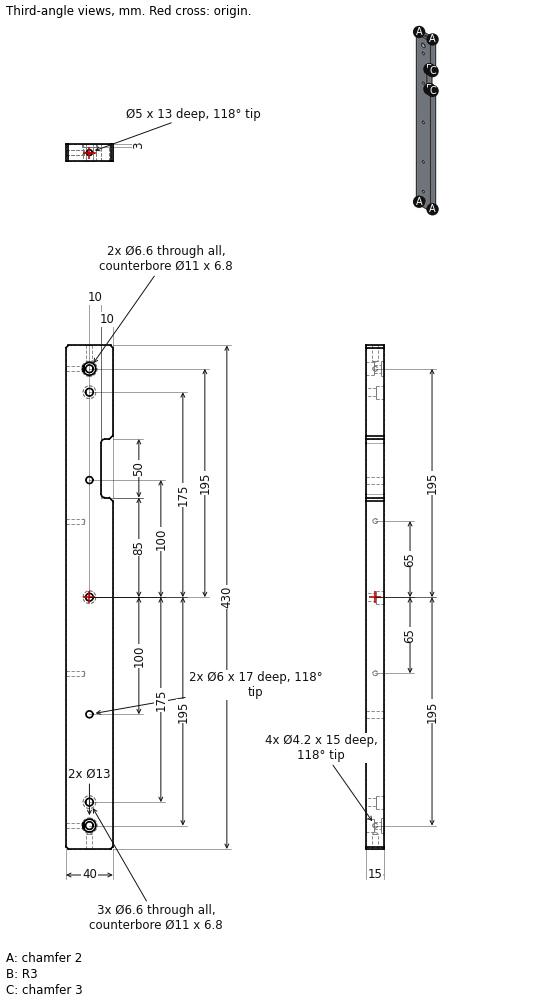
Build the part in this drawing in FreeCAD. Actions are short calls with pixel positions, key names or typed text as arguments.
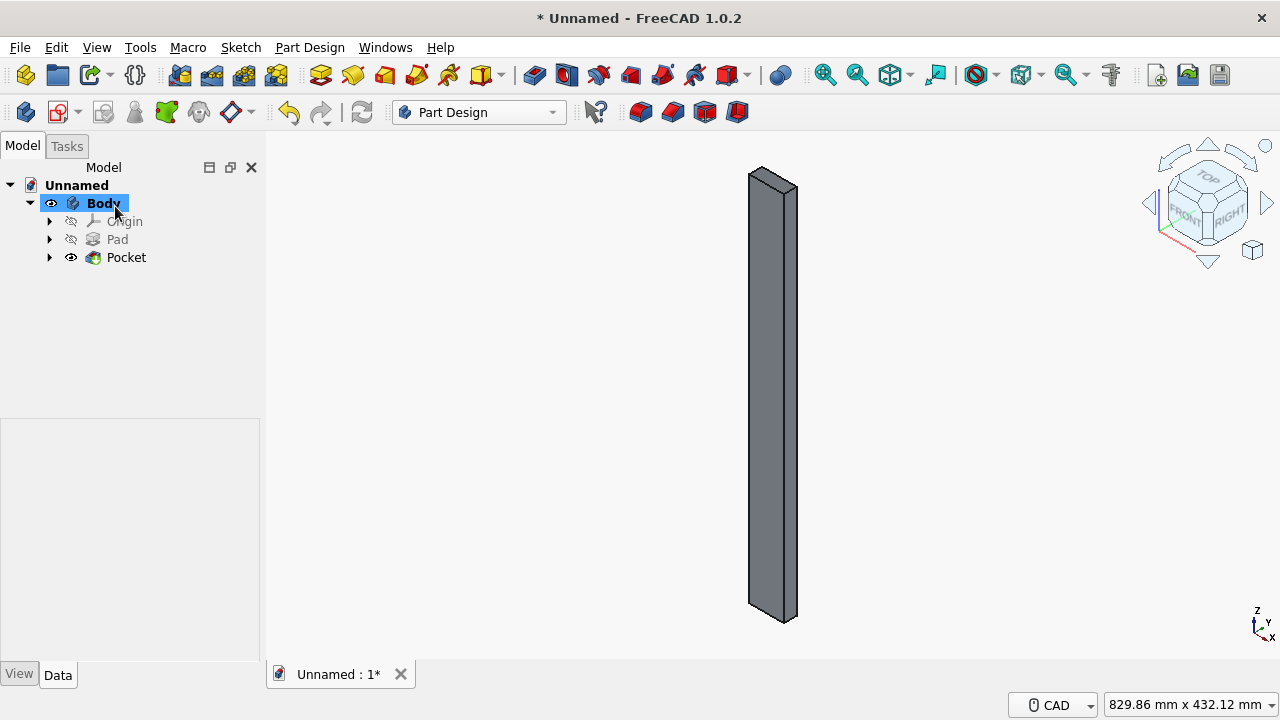
click(767, 214)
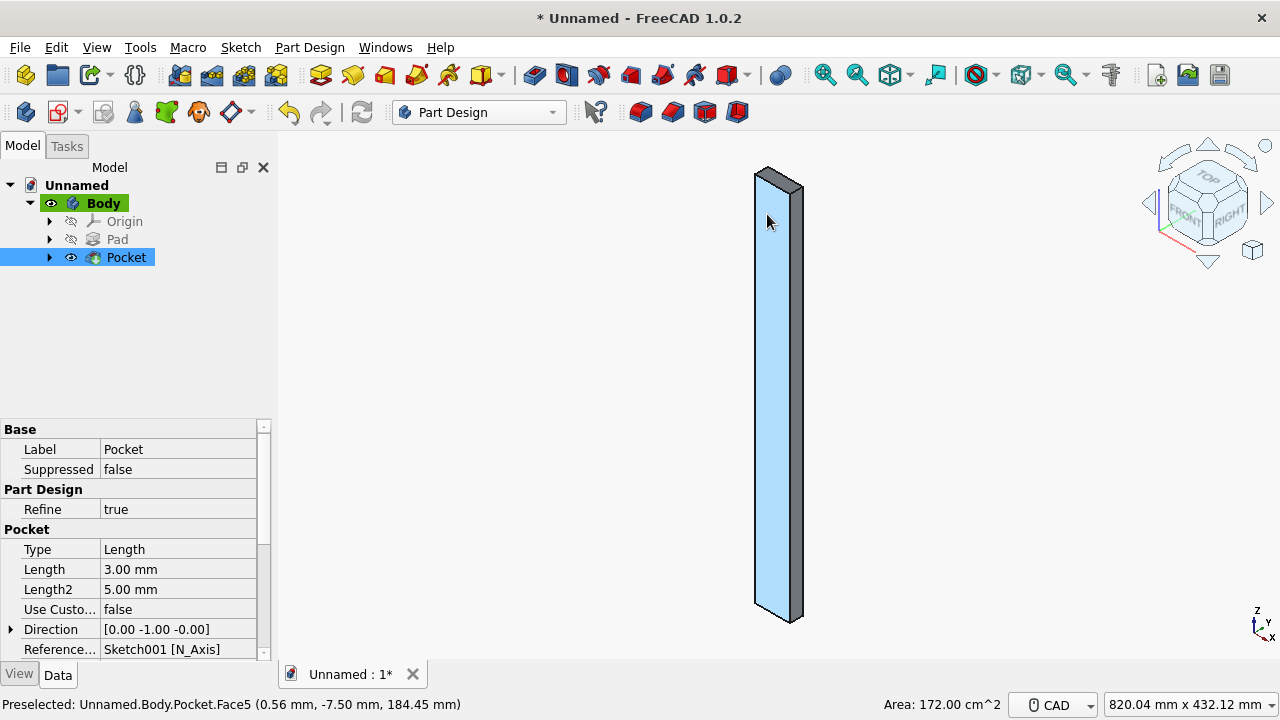
click(58, 112)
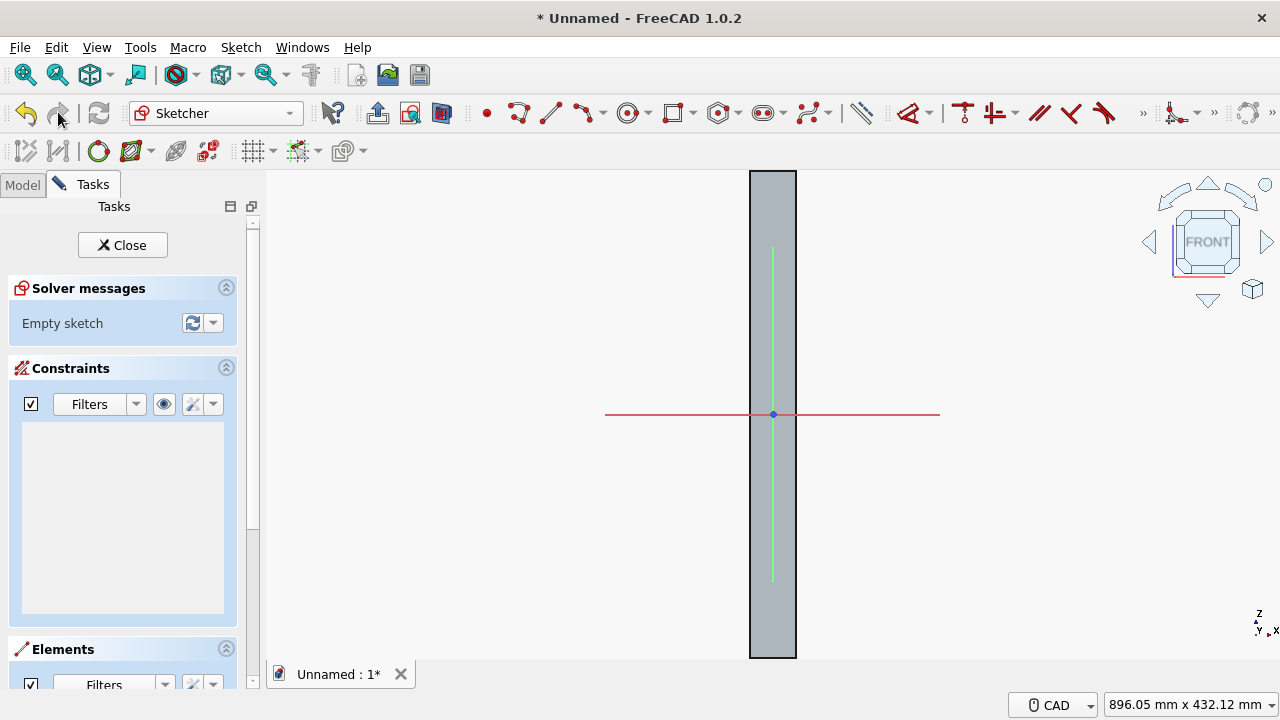
scroll(565, 414, down, 2)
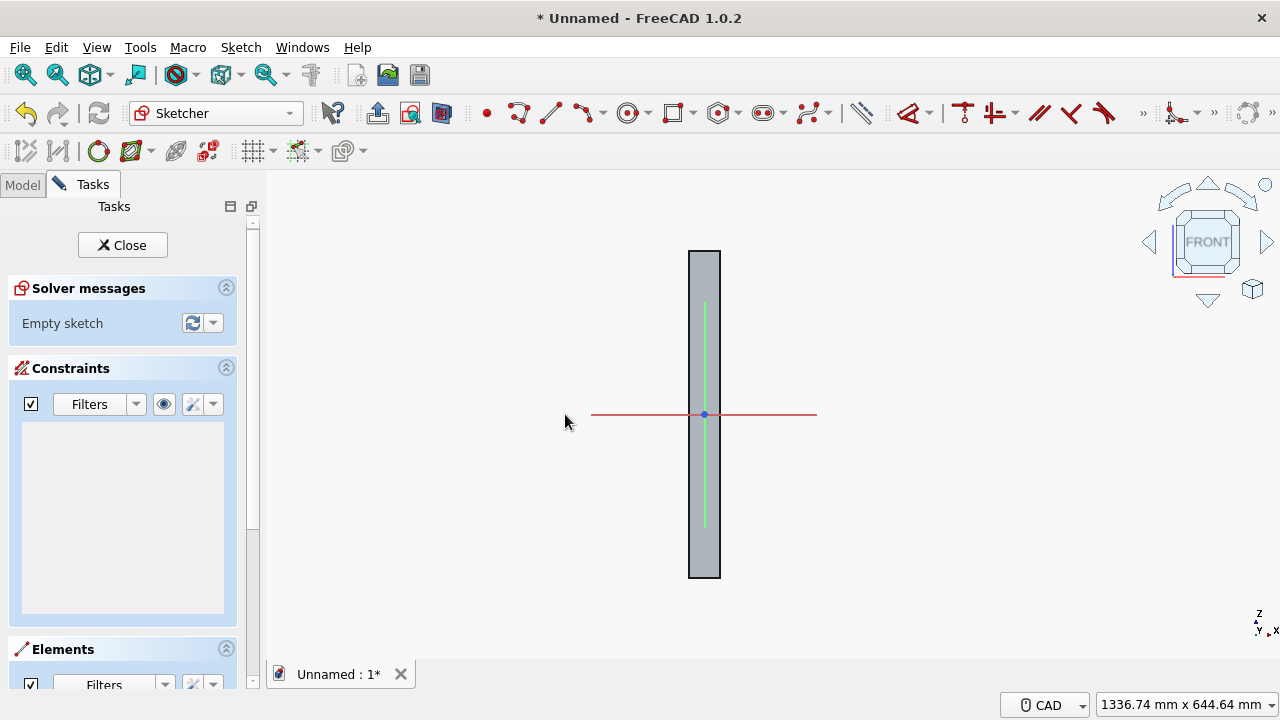
click(628, 114)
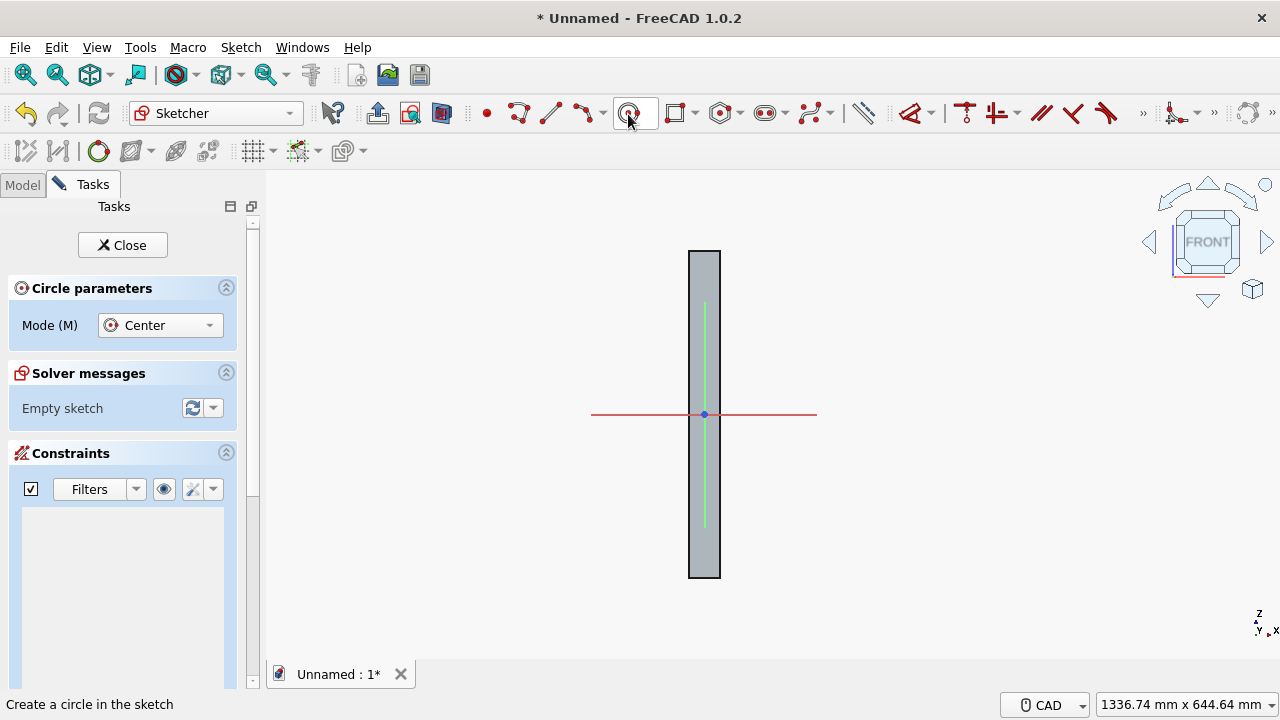
scroll(705, 267, up, 12)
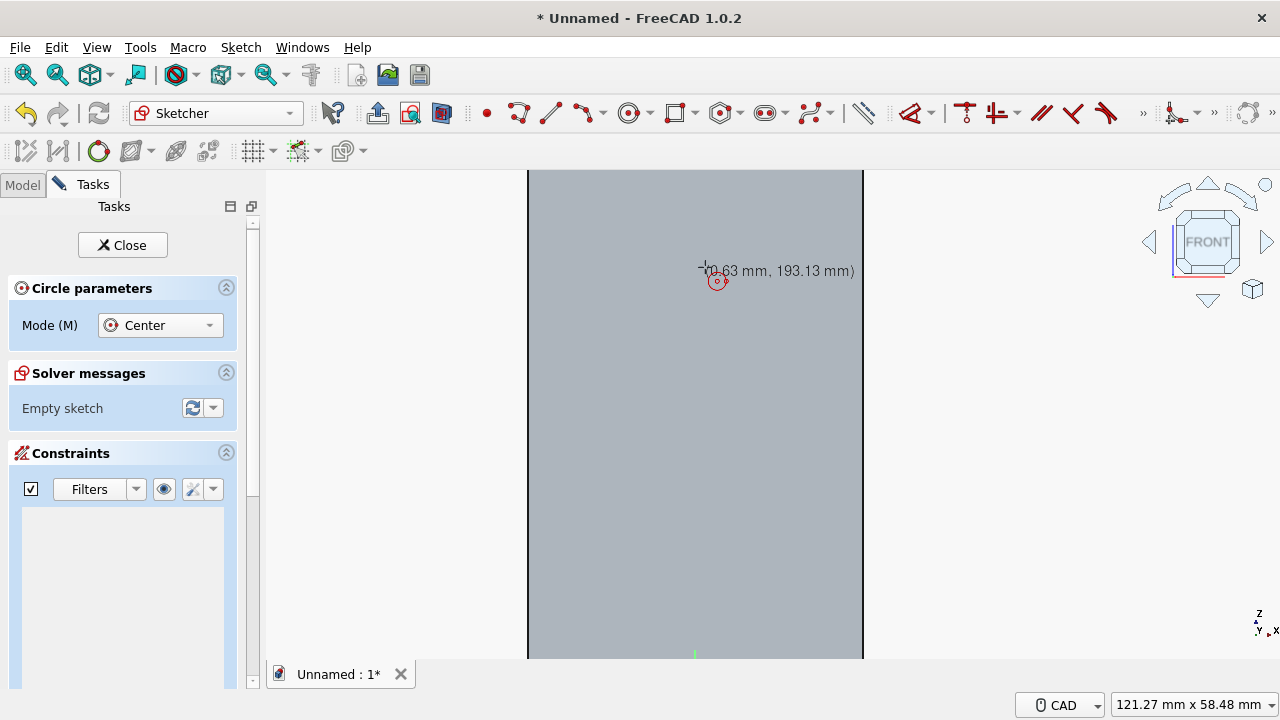
scroll(705, 267, down, 12)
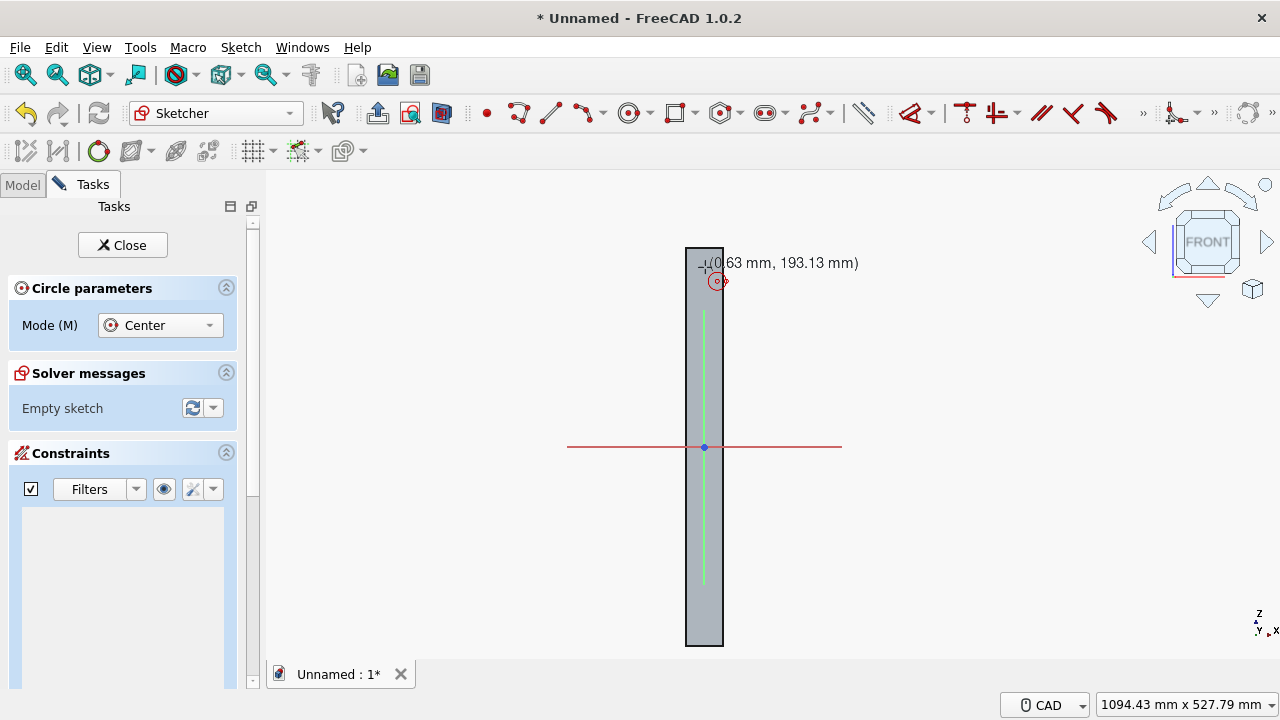
click(705, 267)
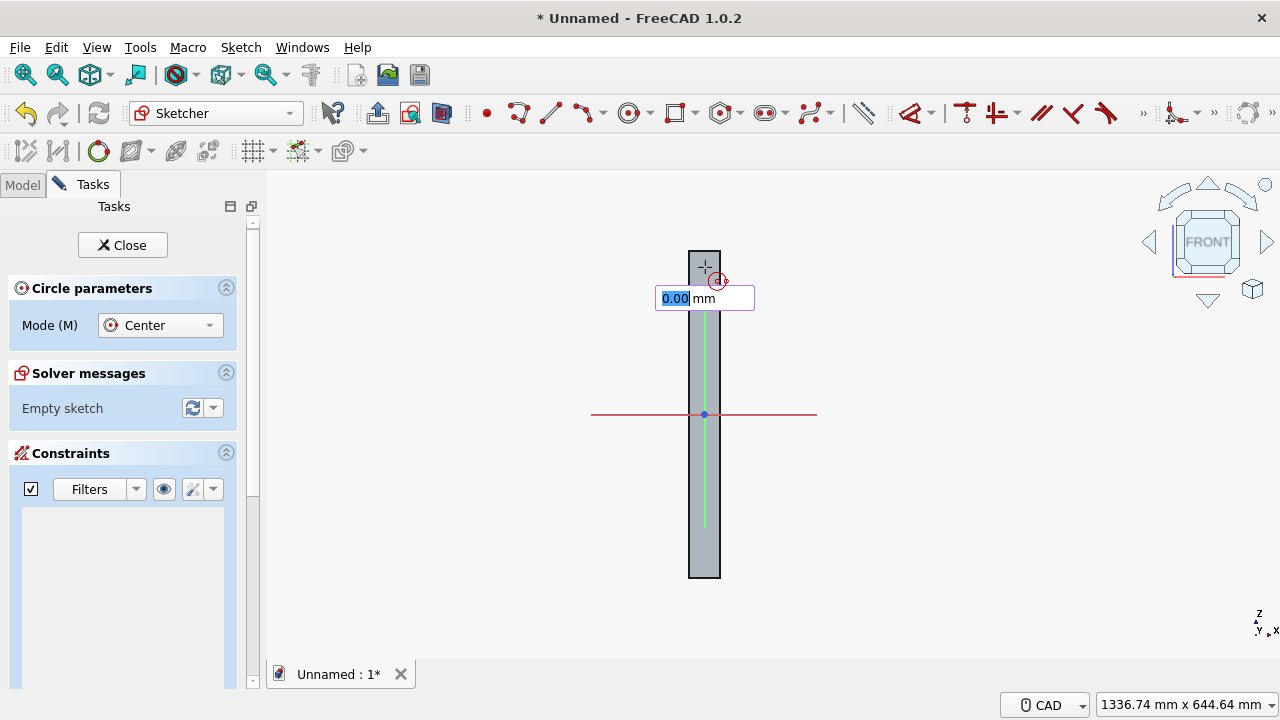
scroll(707, 266, up, 10)
move(703, 263)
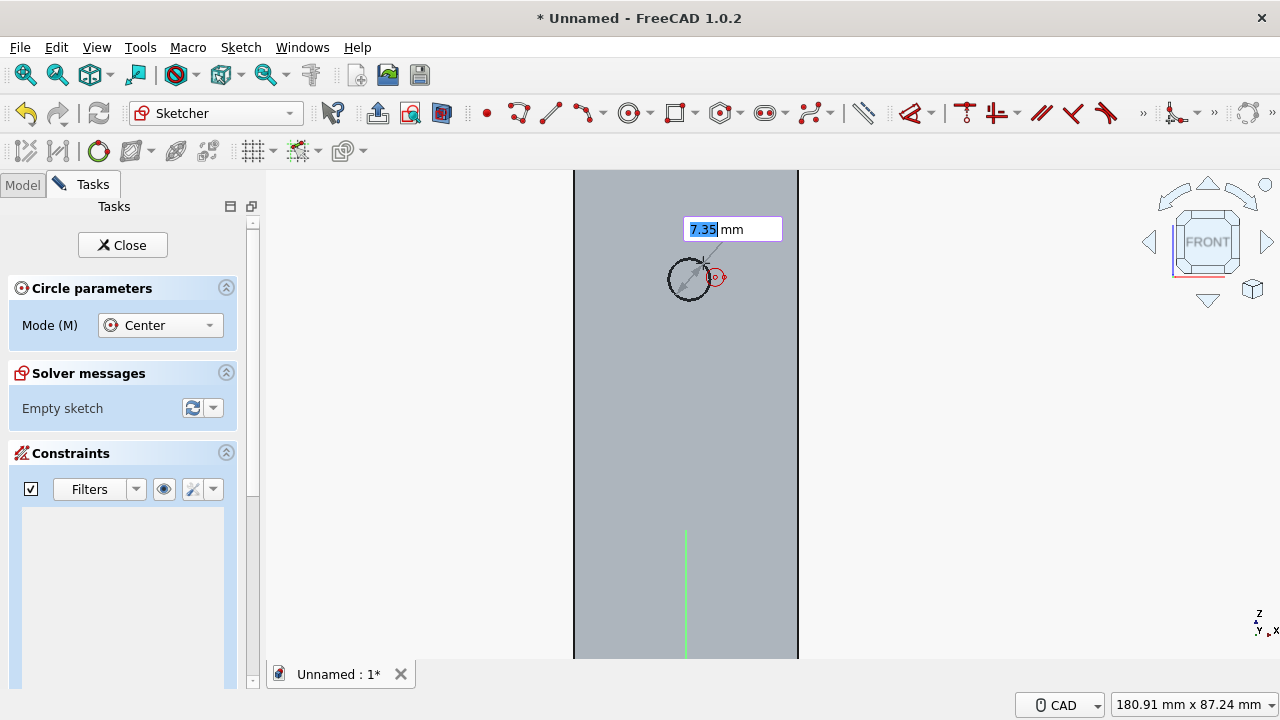
text(6.6)
key(Return)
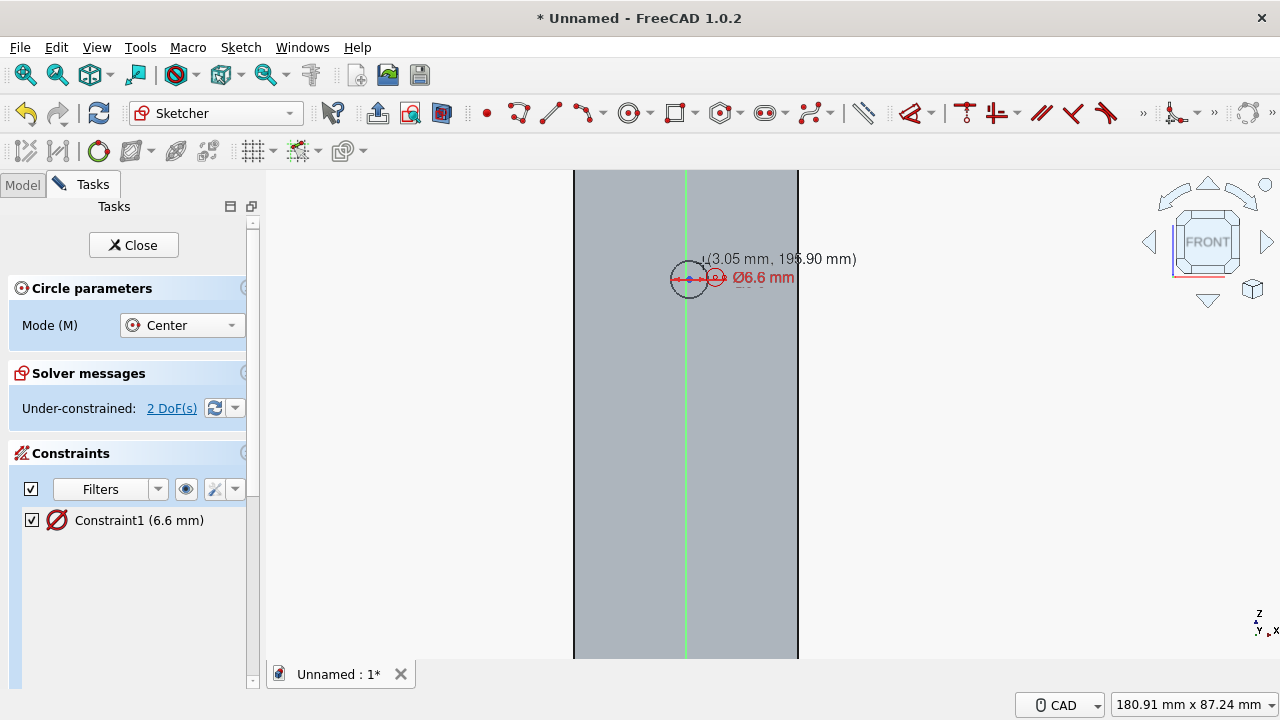
scroll(707, 266, down, 10)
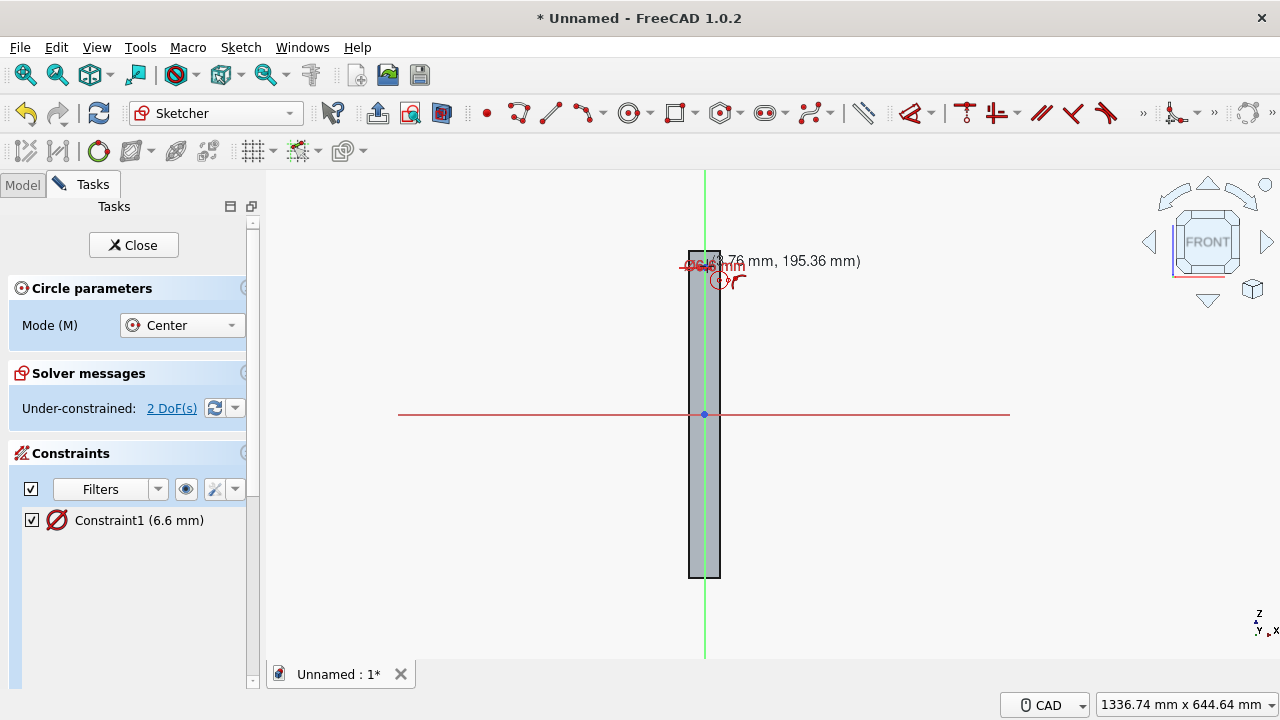
scroll(705, 562, up, 12)